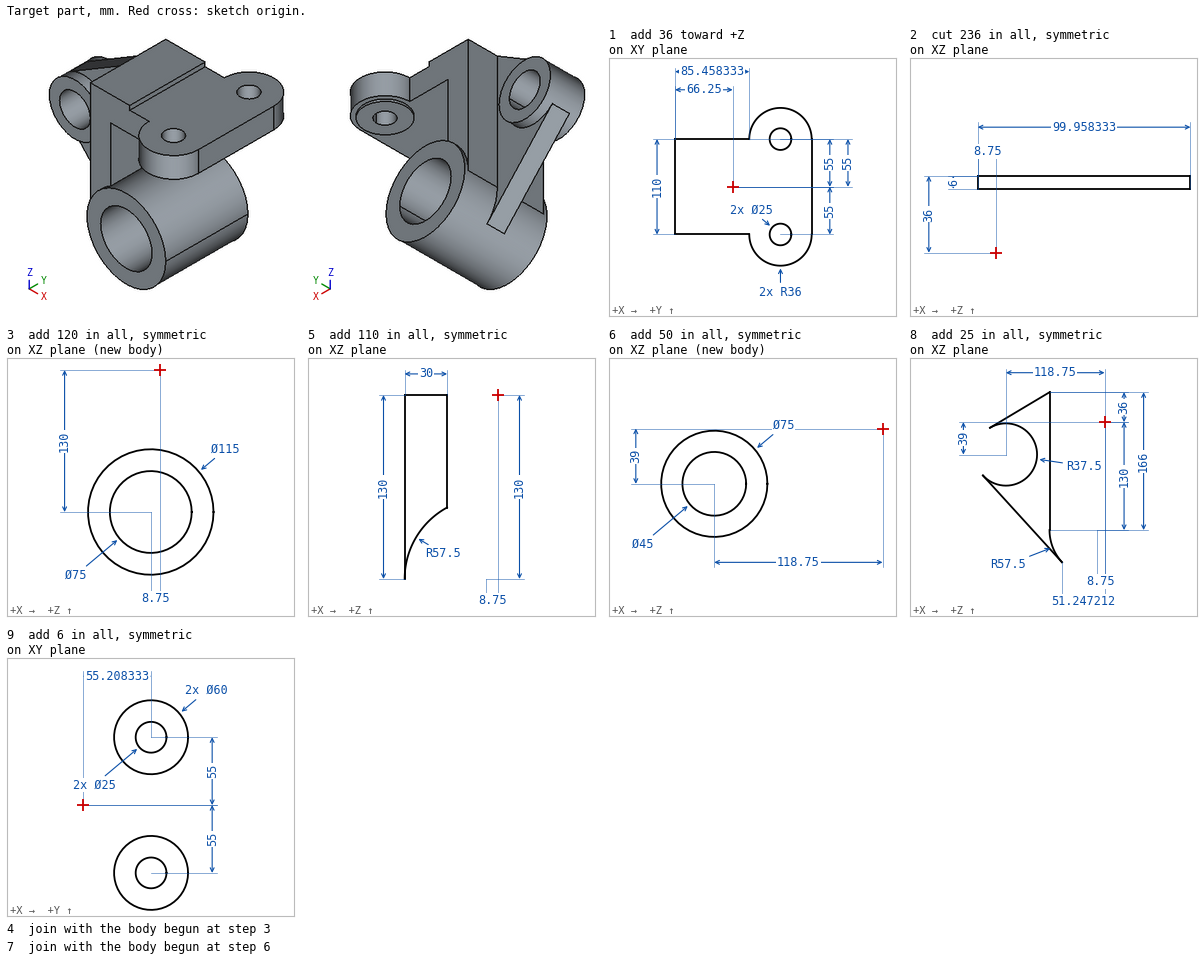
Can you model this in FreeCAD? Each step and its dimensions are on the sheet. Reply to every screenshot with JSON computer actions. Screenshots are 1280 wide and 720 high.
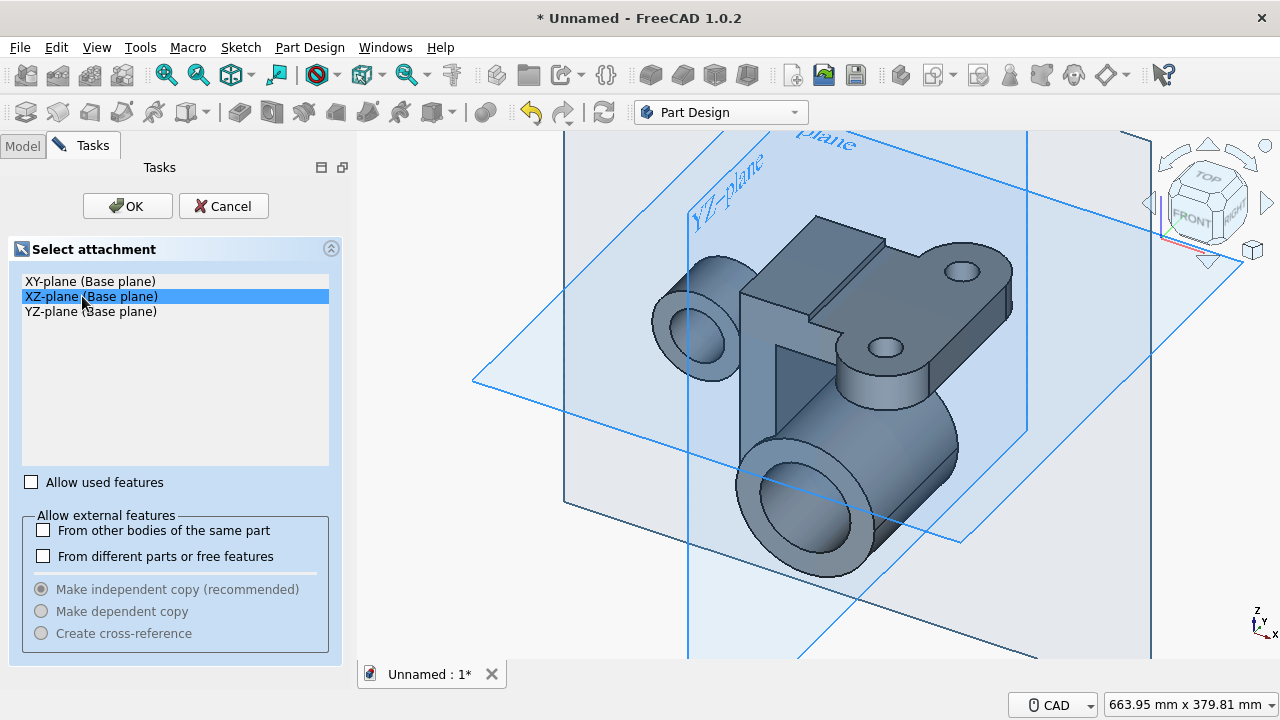
{"action": "left_click", "coordinate": [128, 206]}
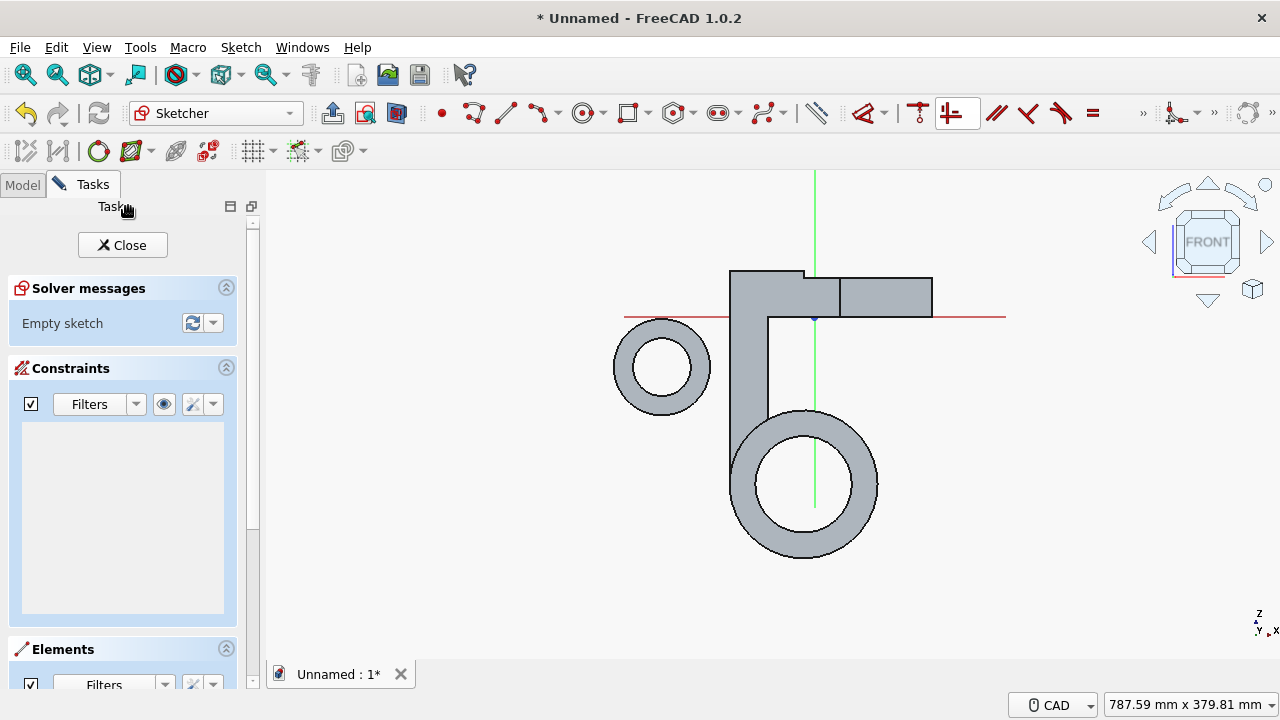
{"action": "left_click", "coordinate": [398, 114]}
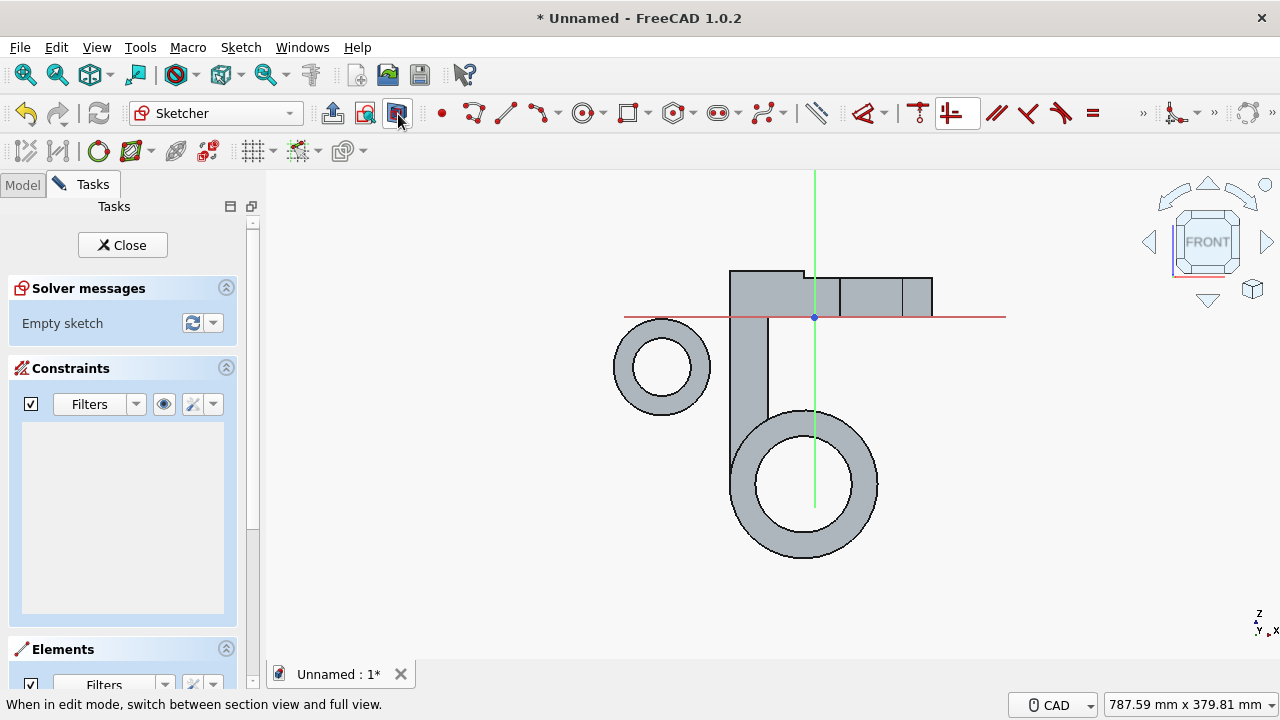
{"action": "left_click", "coordinate": [506, 114]}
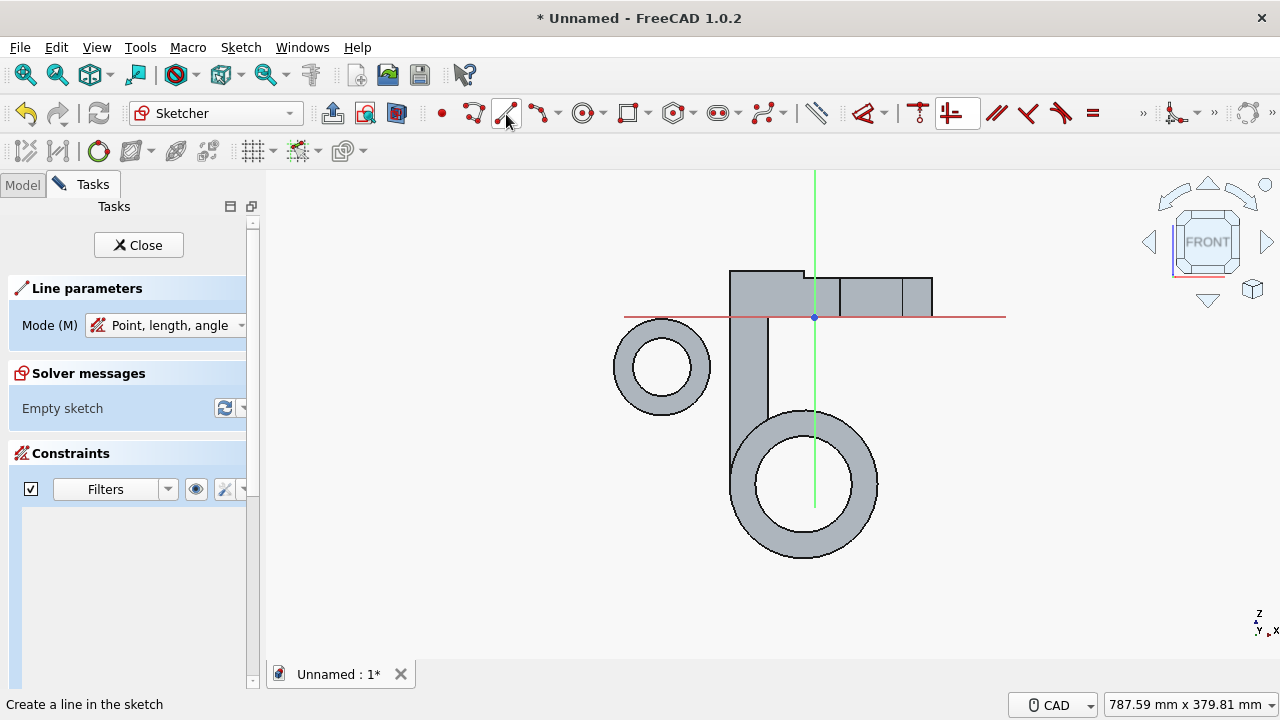
{"action": "left_click", "coordinate": [749, 534]}
{"action": "left_click", "coordinate": [626, 400]}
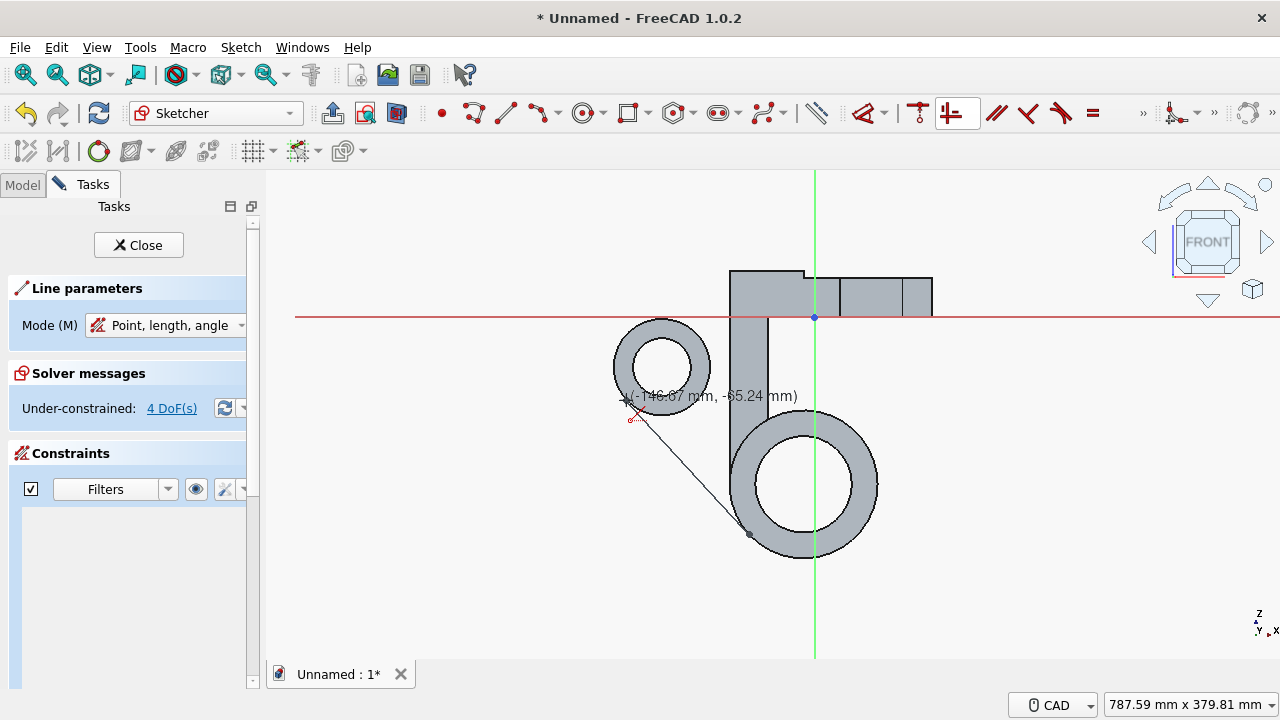
{"action": "left_click", "coordinate": [474, 114]}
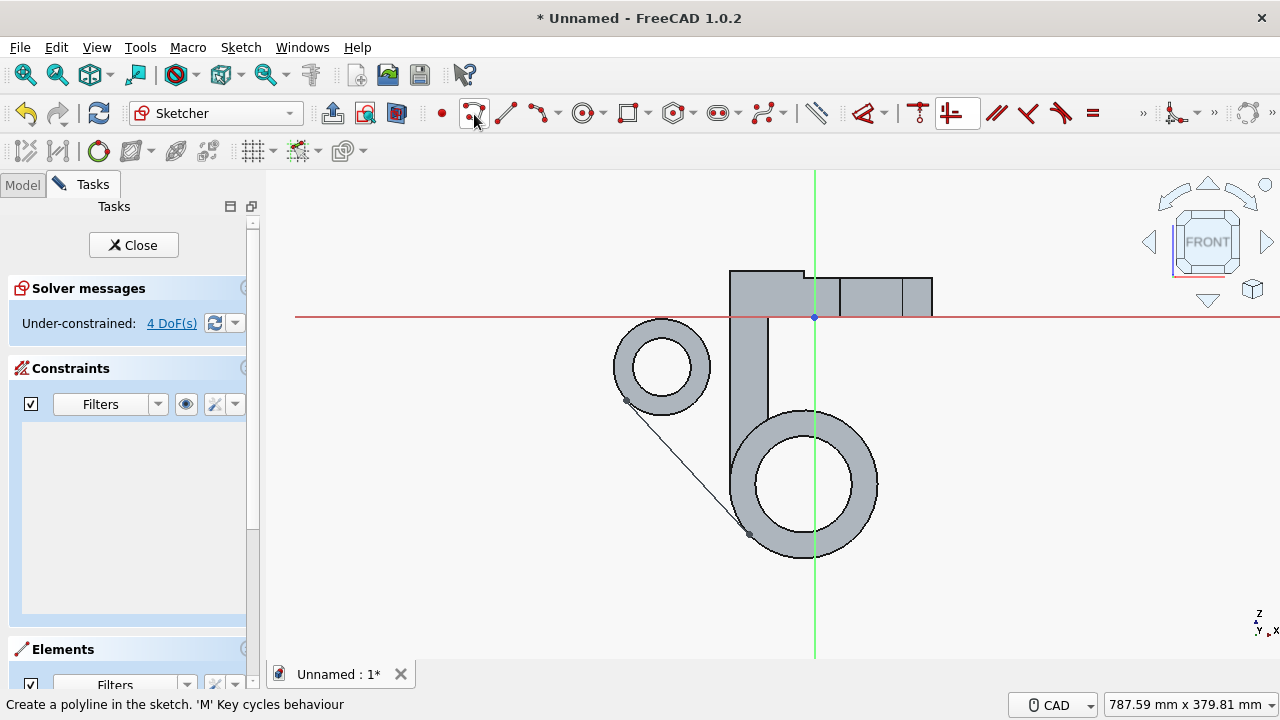
{"action": "scroll", "coordinate": [637, 326], "scroll_direction": "up", "scroll_amount": 3}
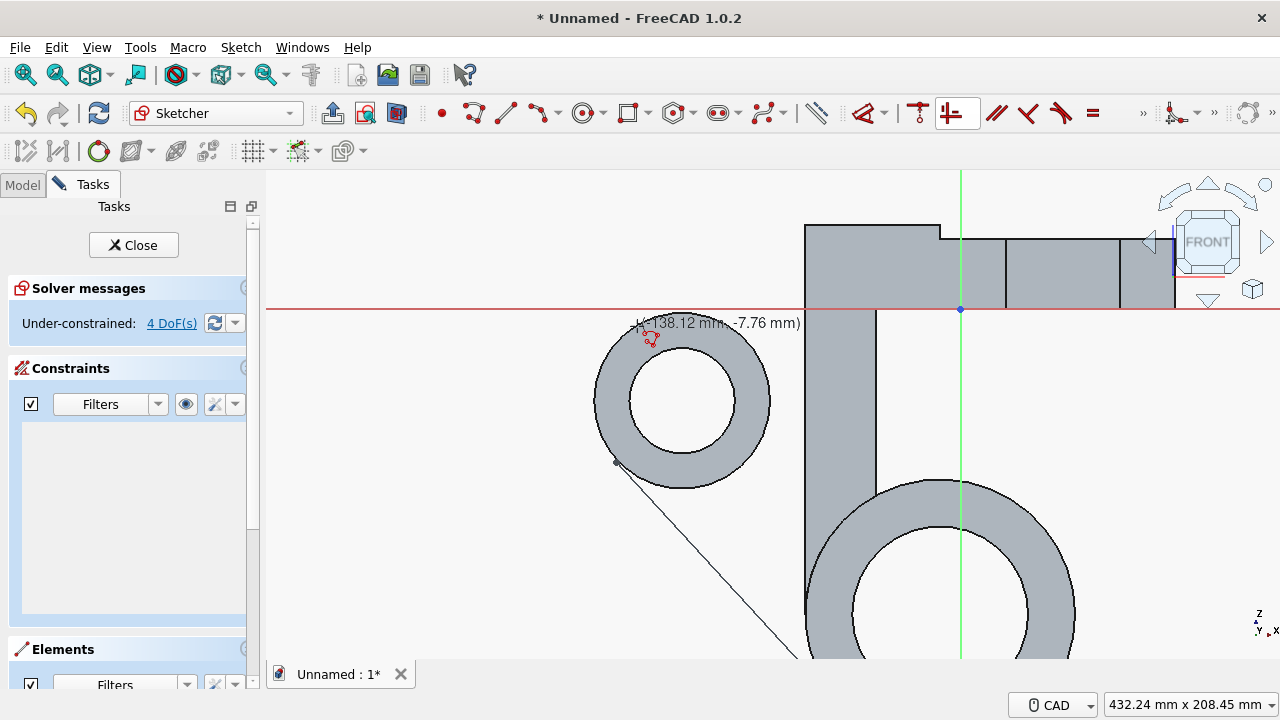
{"action": "left_click", "coordinate": [637, 325]}
{"action": "left_click", "coordinate": [805, 225]}
{"action": "left_click", "coordinate": [805, 614]}
{"action": "right_click", "coordinate": [805, 614]}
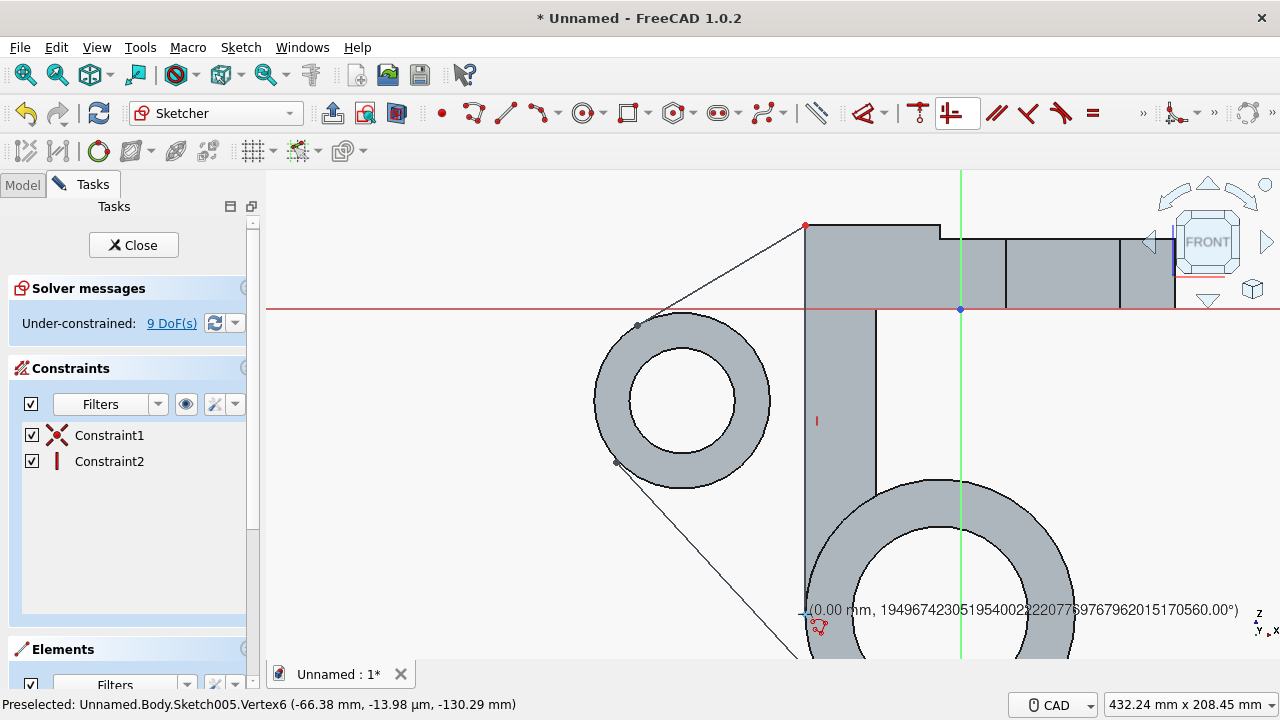
{"action": "left_click", "coordinate": [538, 114]}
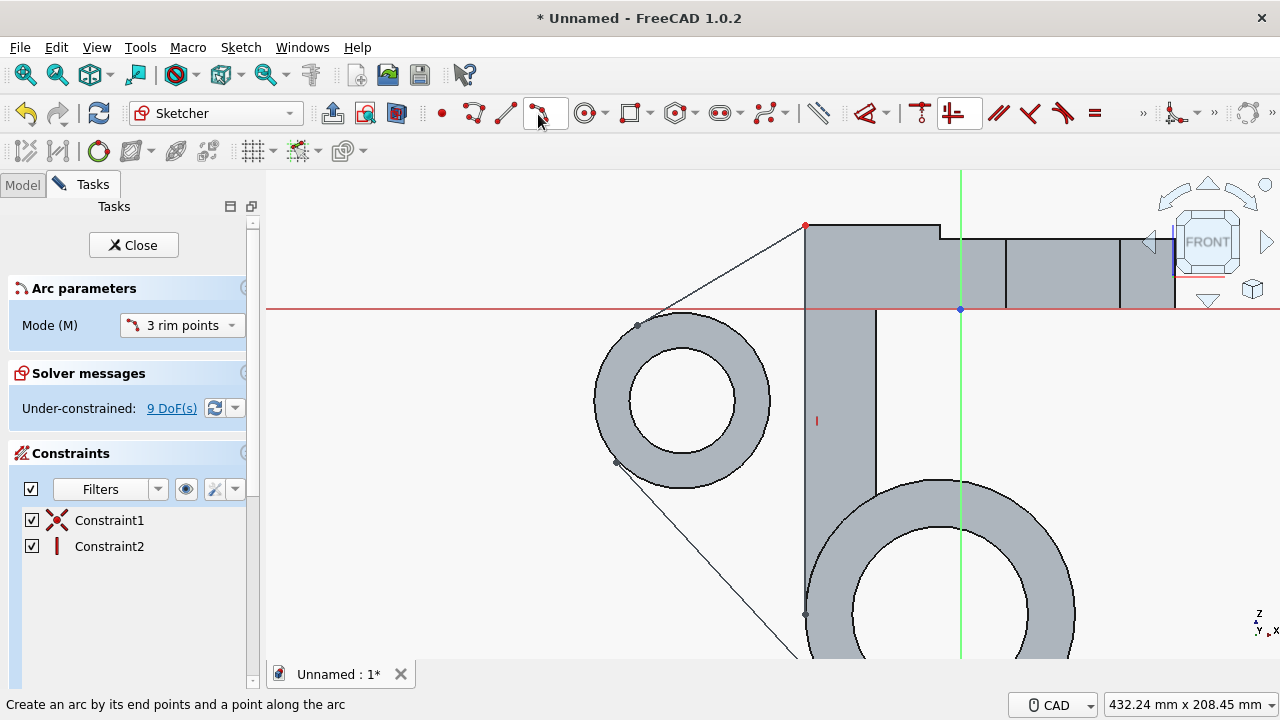
{"action": "left_click", "coordinate": [617, 462]}
{"action": "left_click", "coordinate": [637, 326]}
{"action": "left_click", "coordinate": [769, 414]}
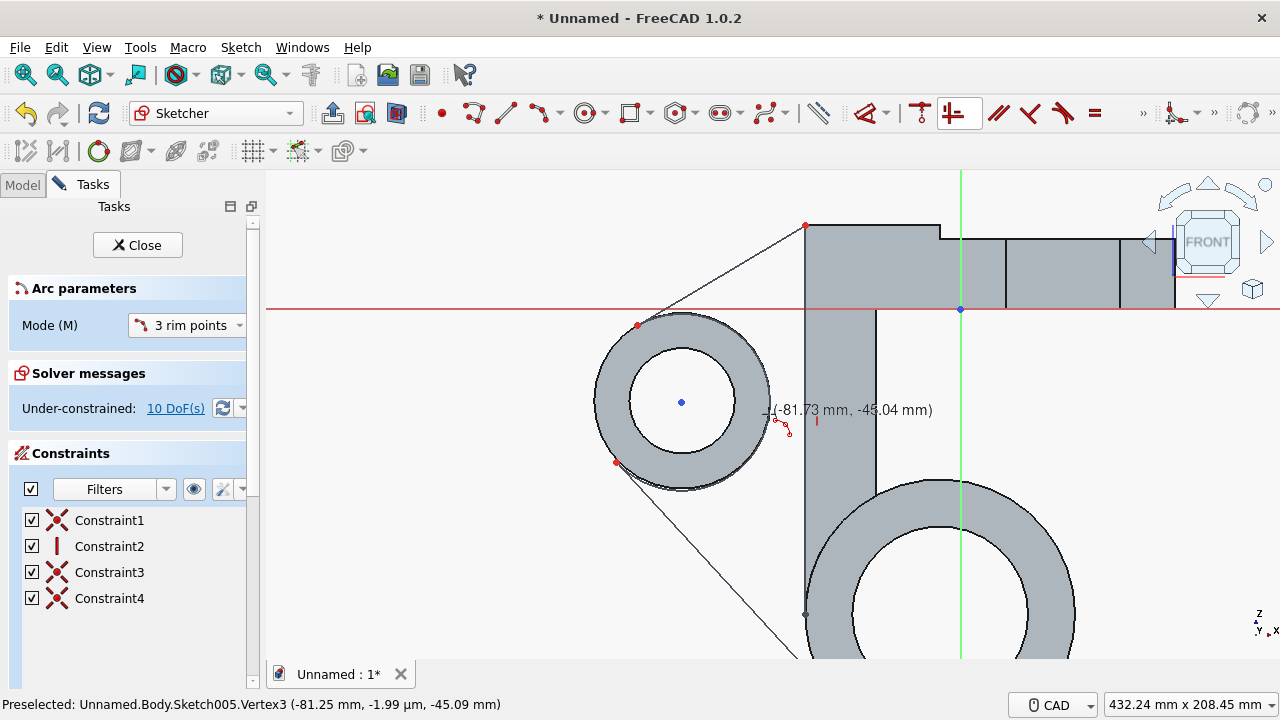
{"action": "left_click", "coordinate": [805, 615]}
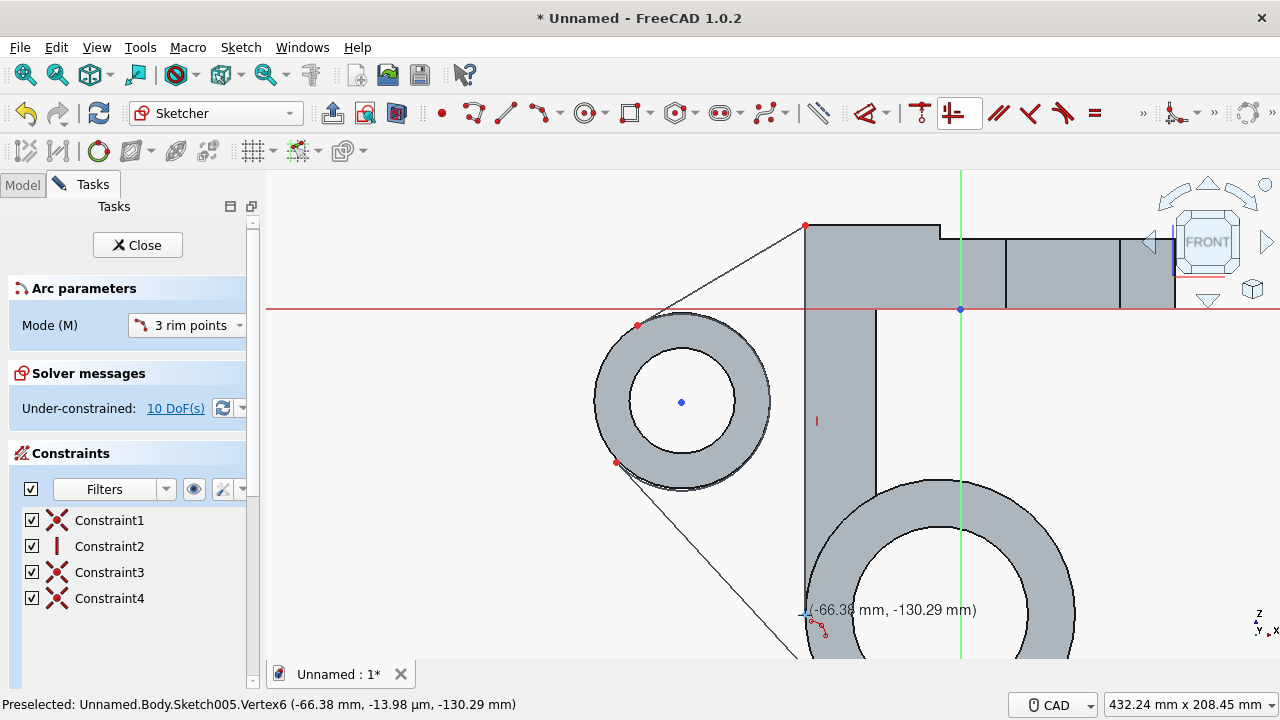
{"action": "scroll", "coordinate": [533, 312], "scroll_direction": "down", "scroll_amount": 2}